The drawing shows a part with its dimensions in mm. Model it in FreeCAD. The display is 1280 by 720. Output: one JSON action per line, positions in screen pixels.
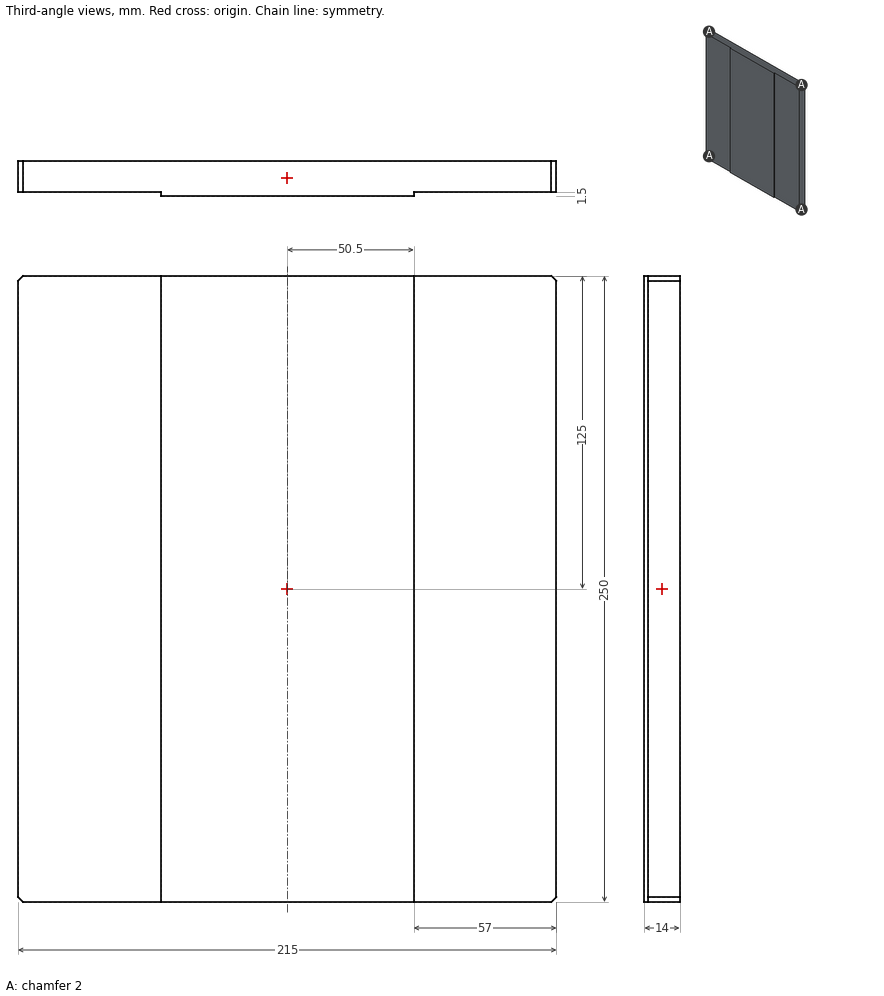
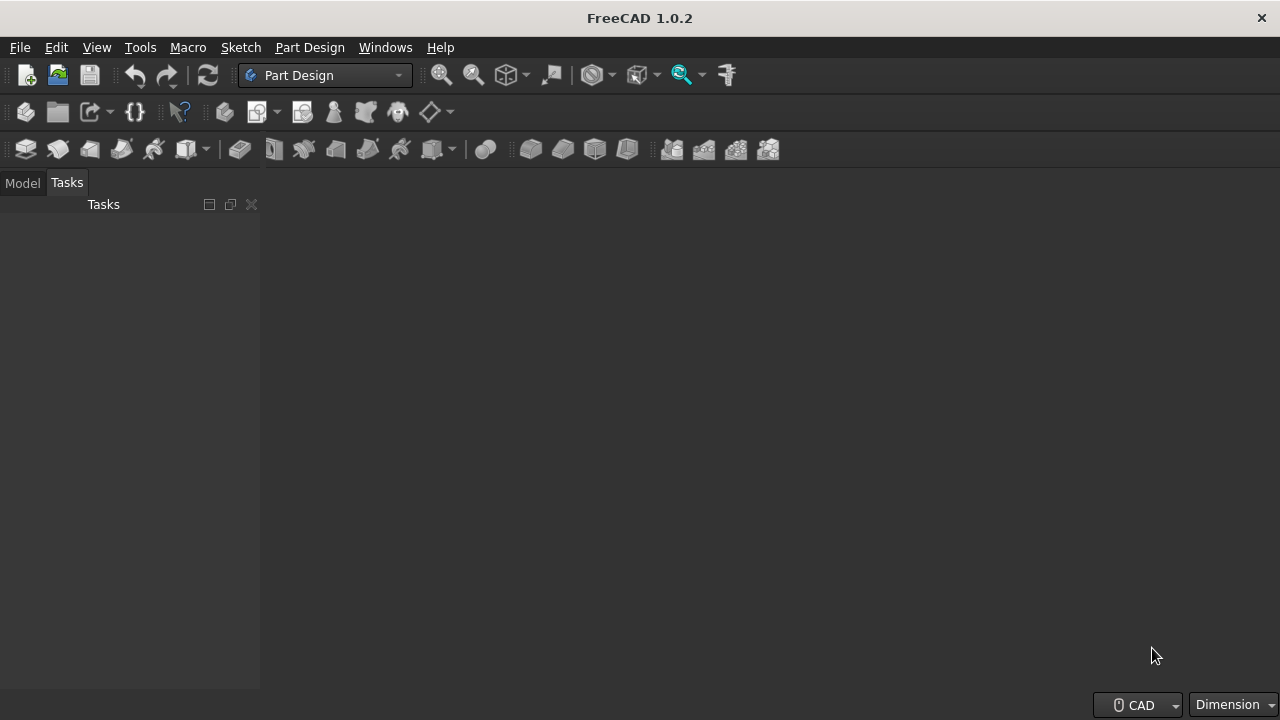
{"action": "key", "text": "ctrl+n"}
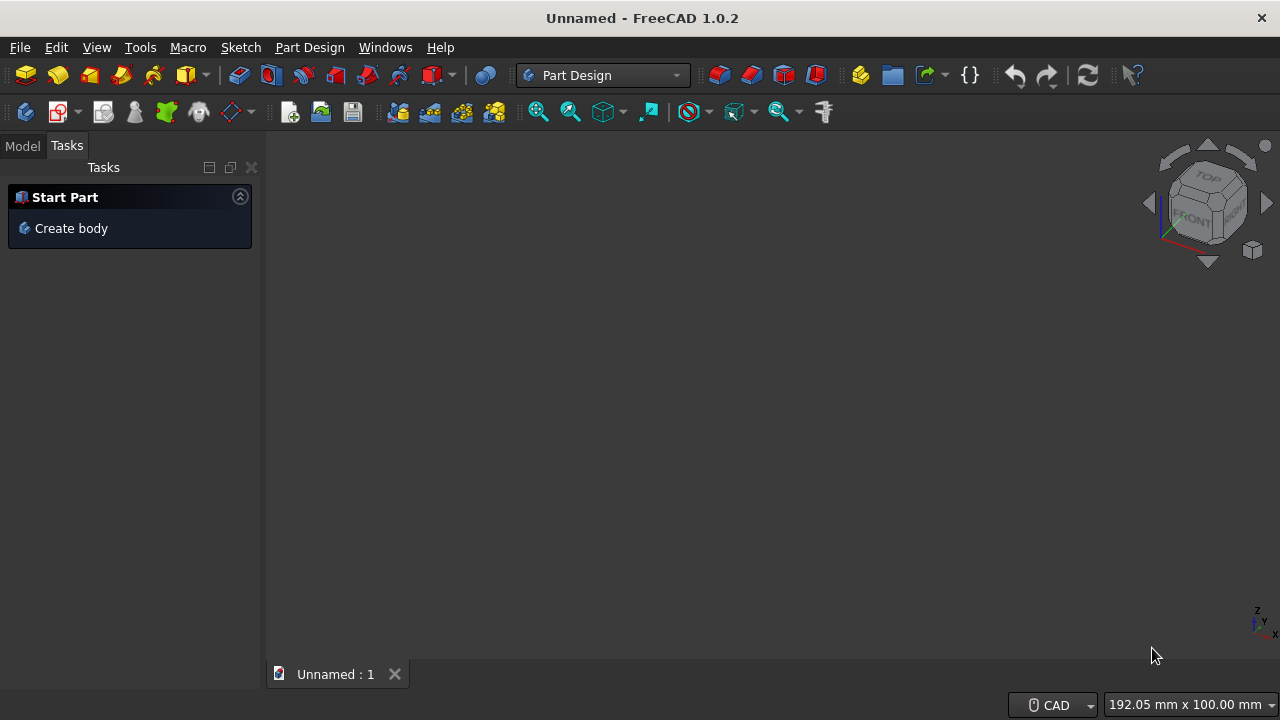
{"action": "left_click", "coordinate": [58, 112]}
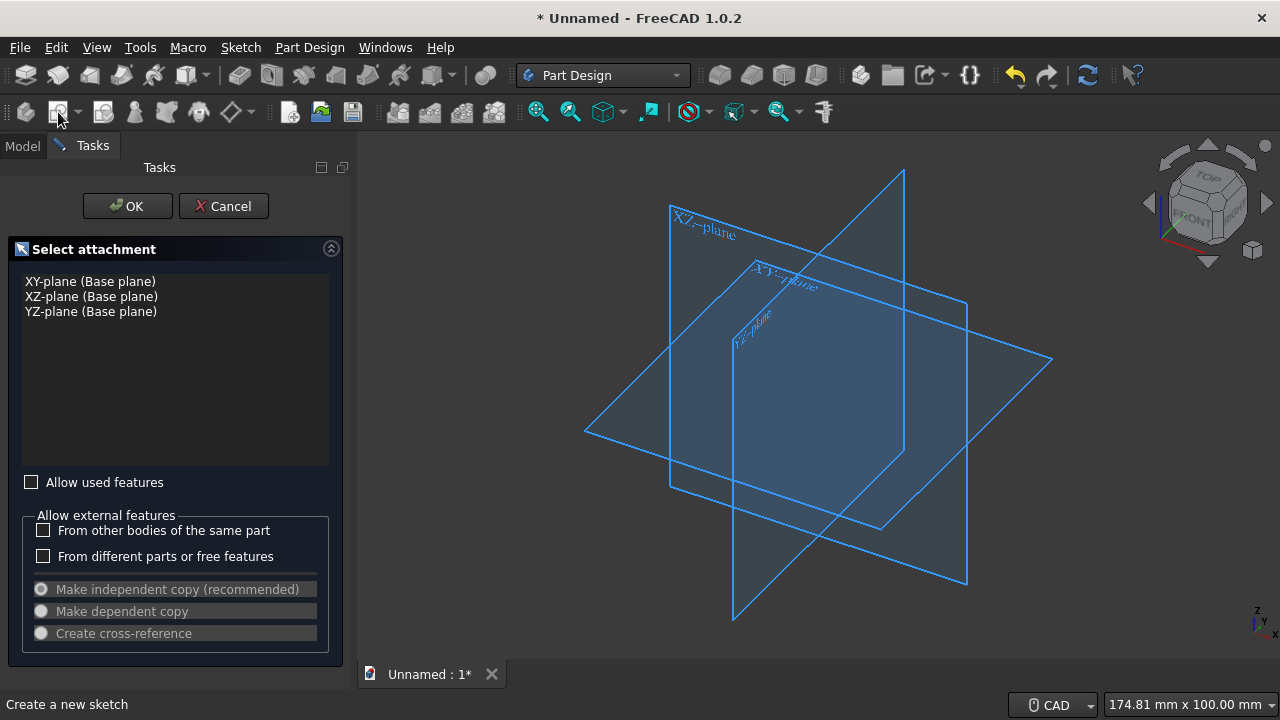
{"action": "left_click", "coordinate": [82, 296]}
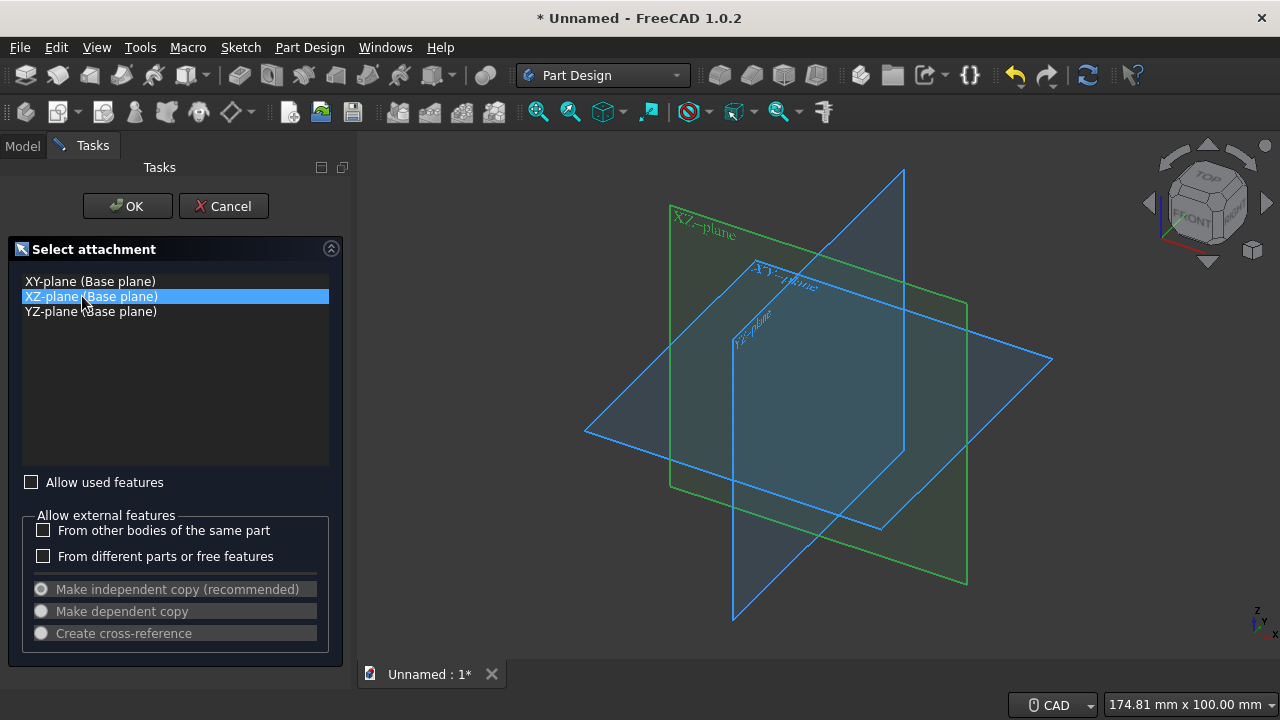
{"action": "left_click", "coordinate": [128, 206]}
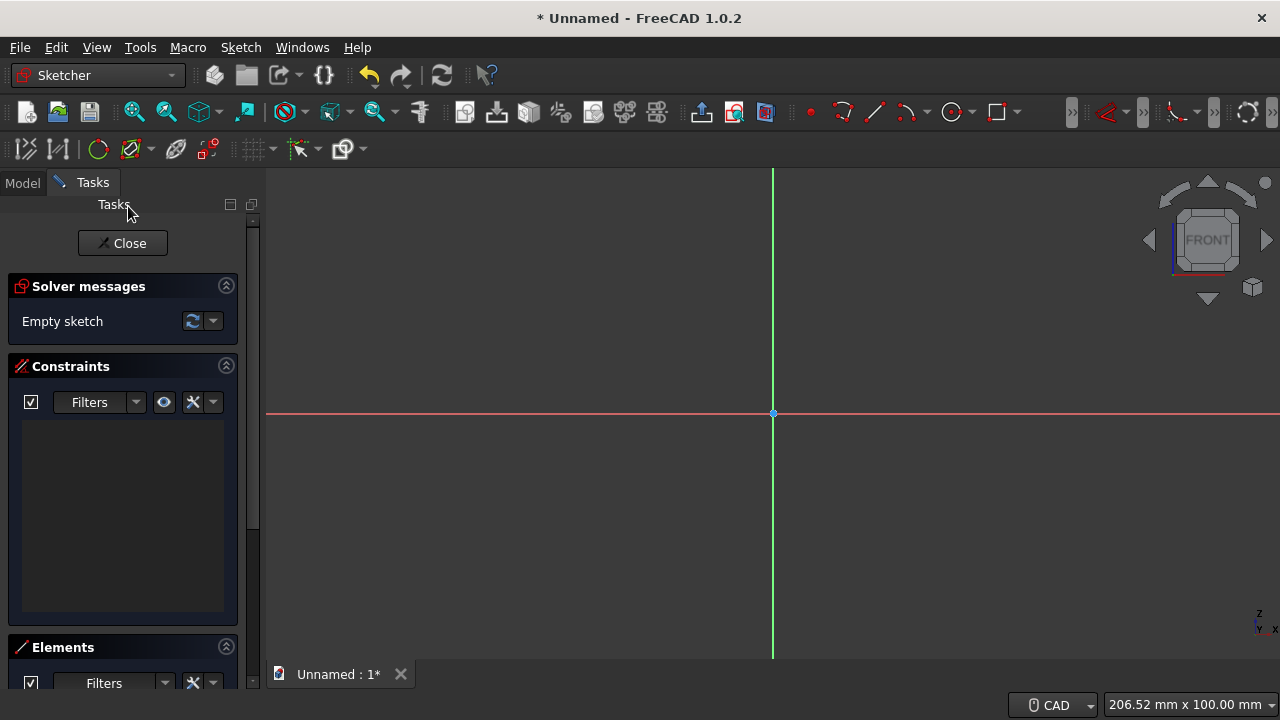
{"action": "scroll", "coordinate": [682, 414], "scroll_direction": "down", "scroll_amount": 7}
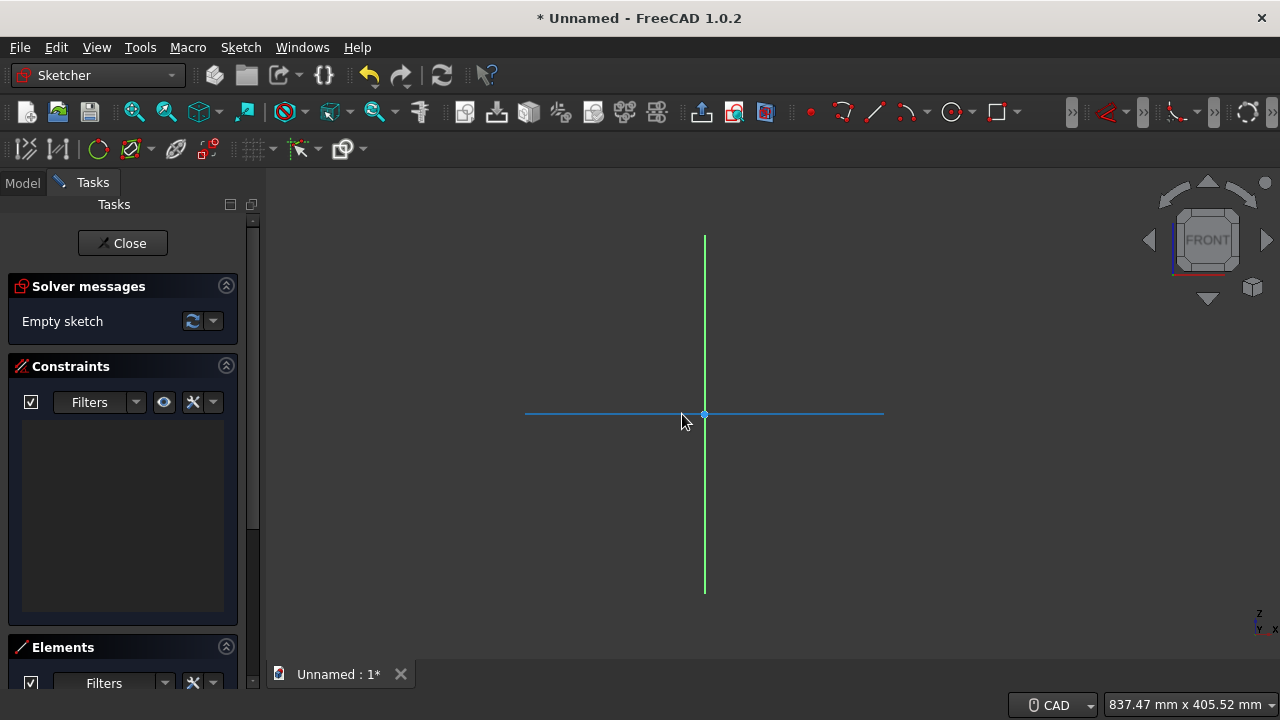
{"action": "key", "text": "g v"}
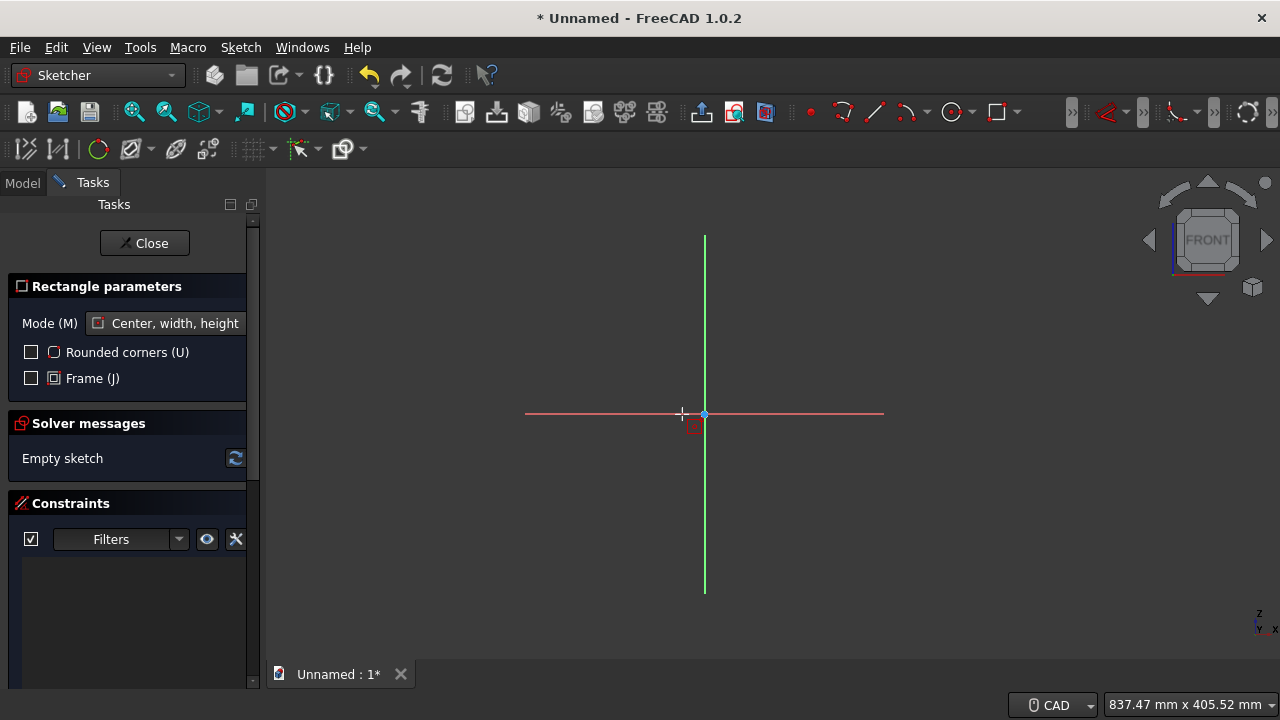
{"action": "left_click", "coordinate": [705, 414]}
{"action": "left_click", "coordinate": [835, 263]}
{"action": "key", "text": "Escape"}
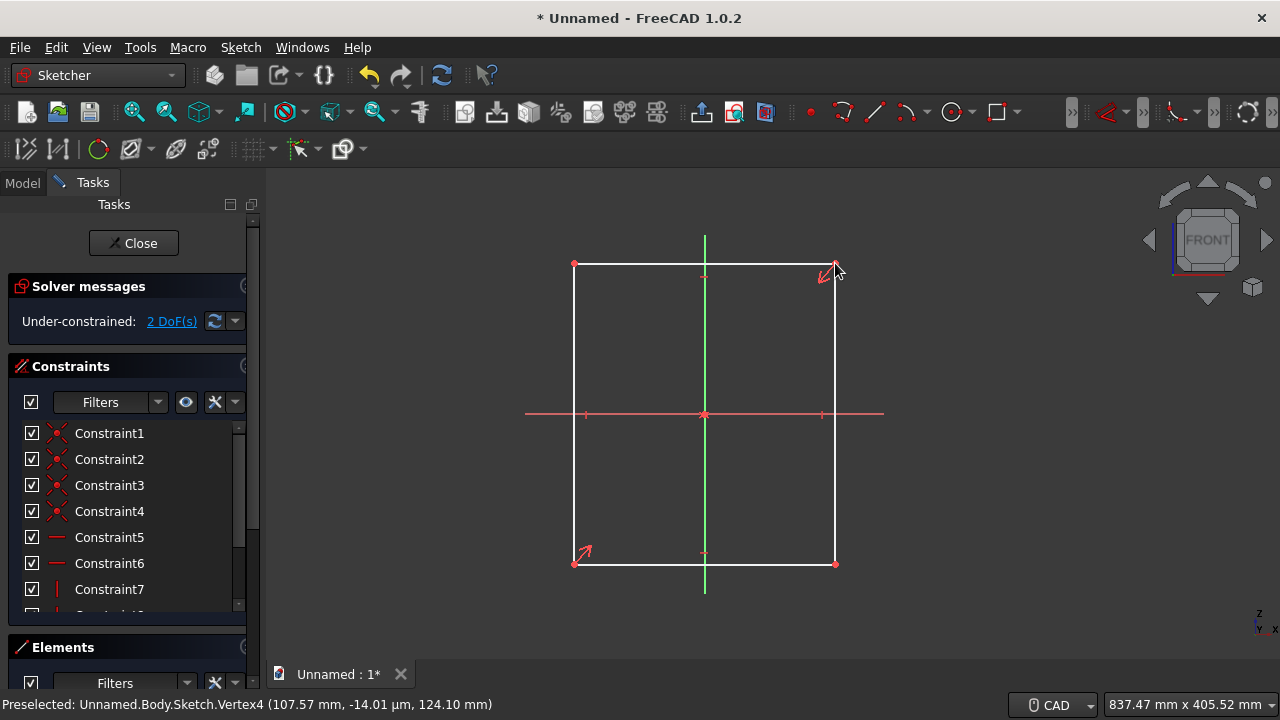
{"action": "left_click", "coordinate": [653, 565]}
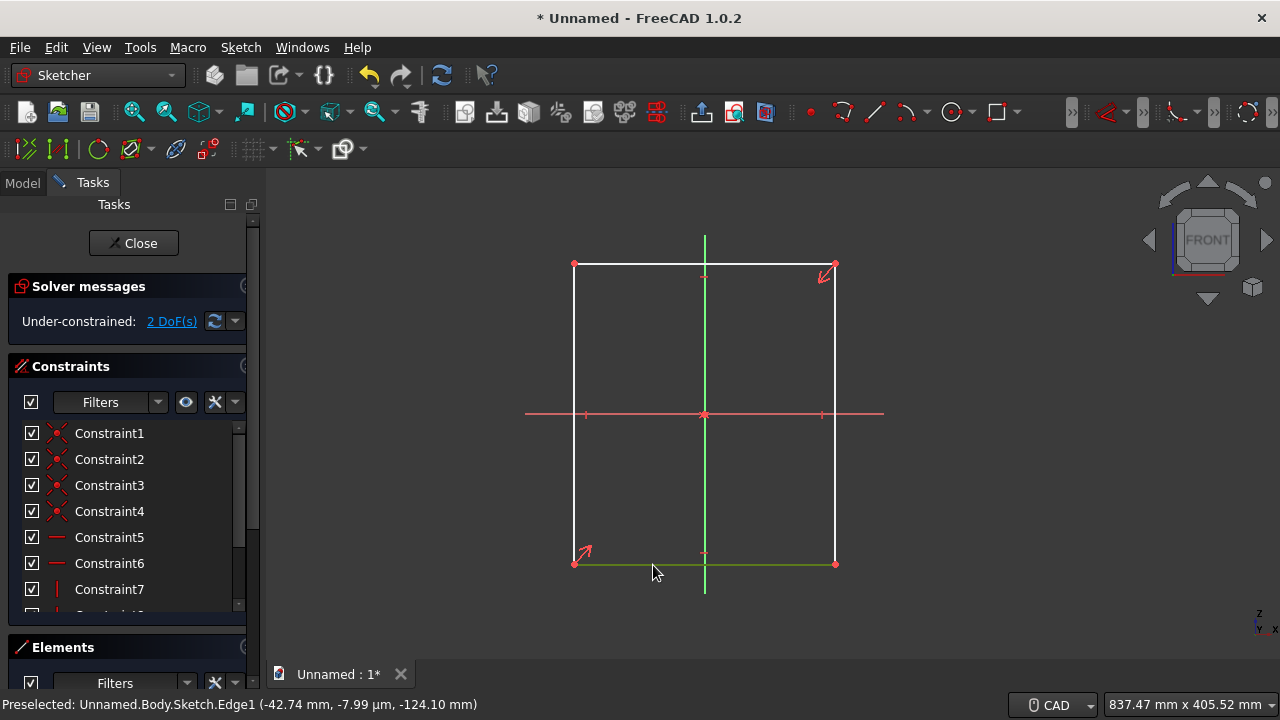
{"action": "key", "text": "l"}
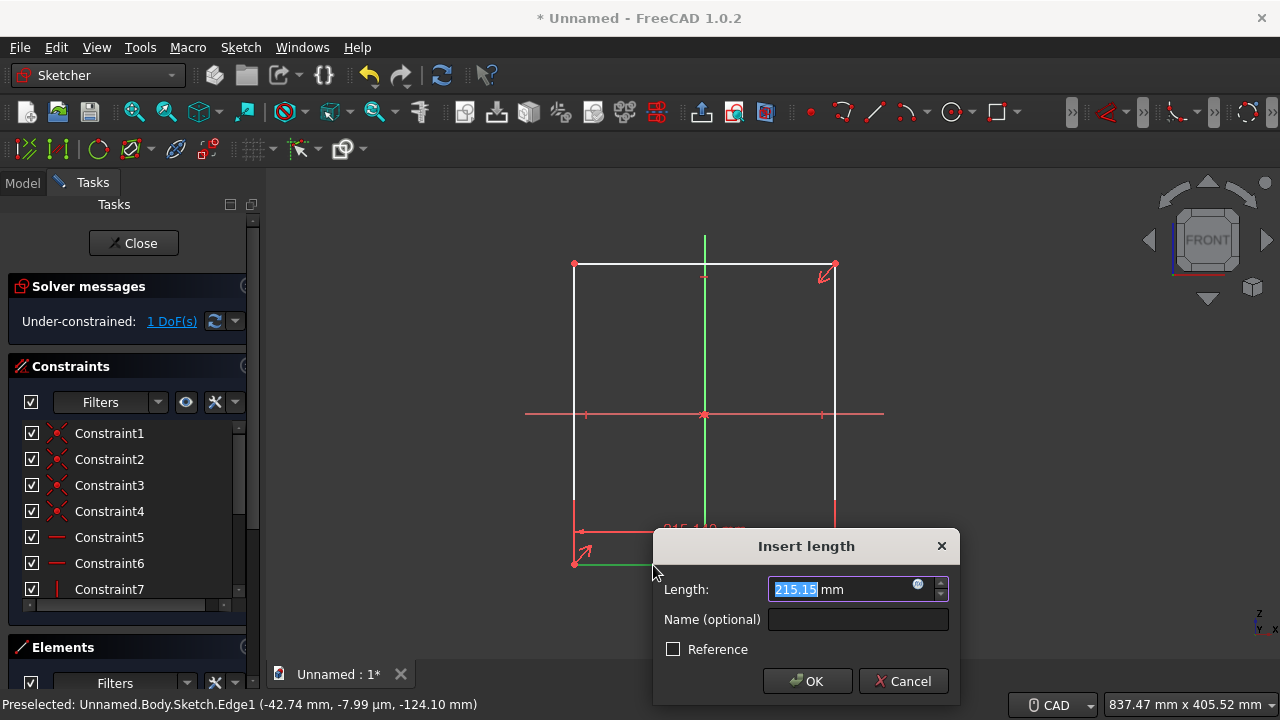
{"action": "type", "text": "215"}
{"action": "key", "text": "Return"}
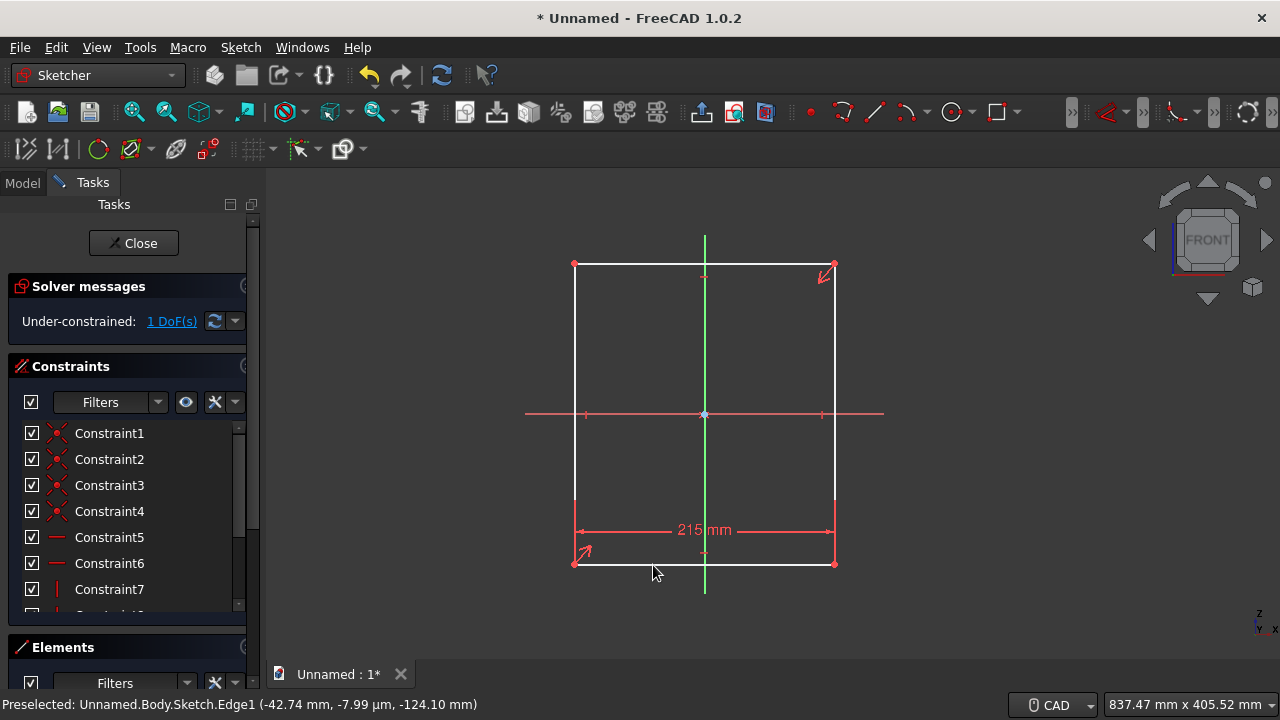
{"action": "left_click", "coordinate": [835, 474]}